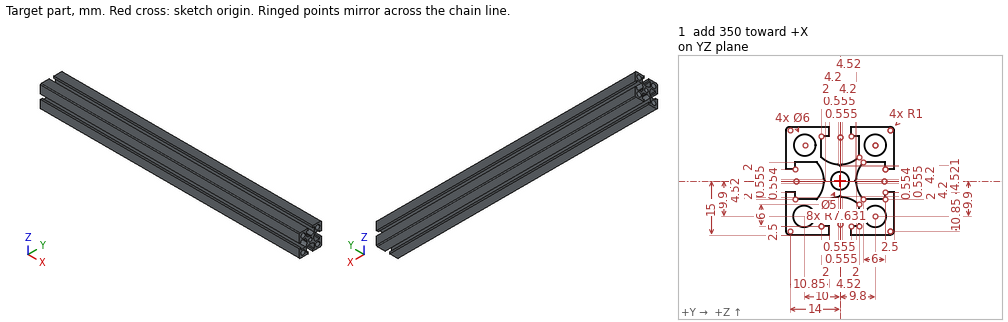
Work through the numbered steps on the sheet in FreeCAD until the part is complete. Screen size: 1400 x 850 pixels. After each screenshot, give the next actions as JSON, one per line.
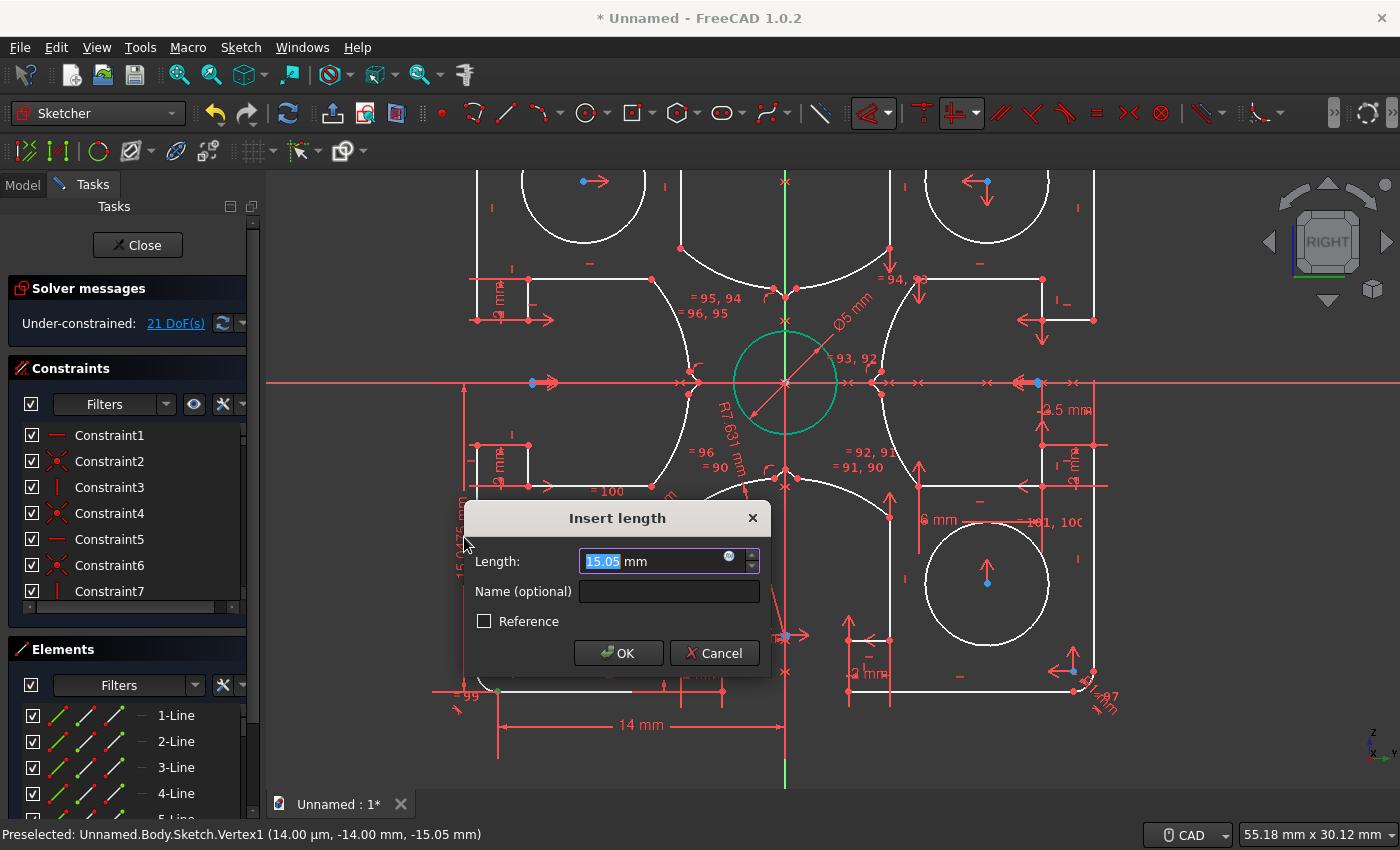
{"action": "type", "text": "15"}
{"action": "key", "text": "Return"}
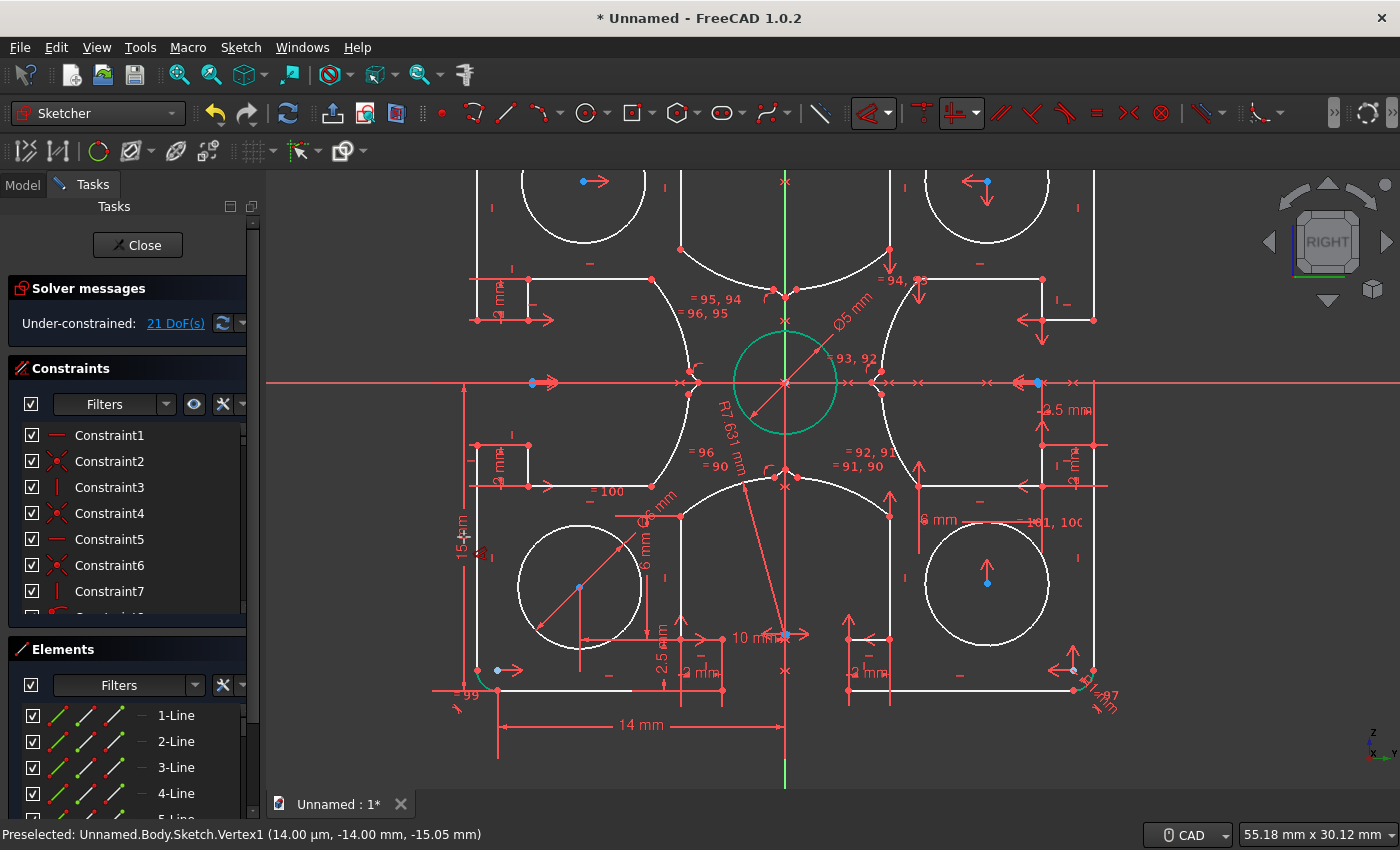
{"action": "left_click", "coordinate": [580, 587]}
{"action": "left_click", "coordinate": [546, 438]}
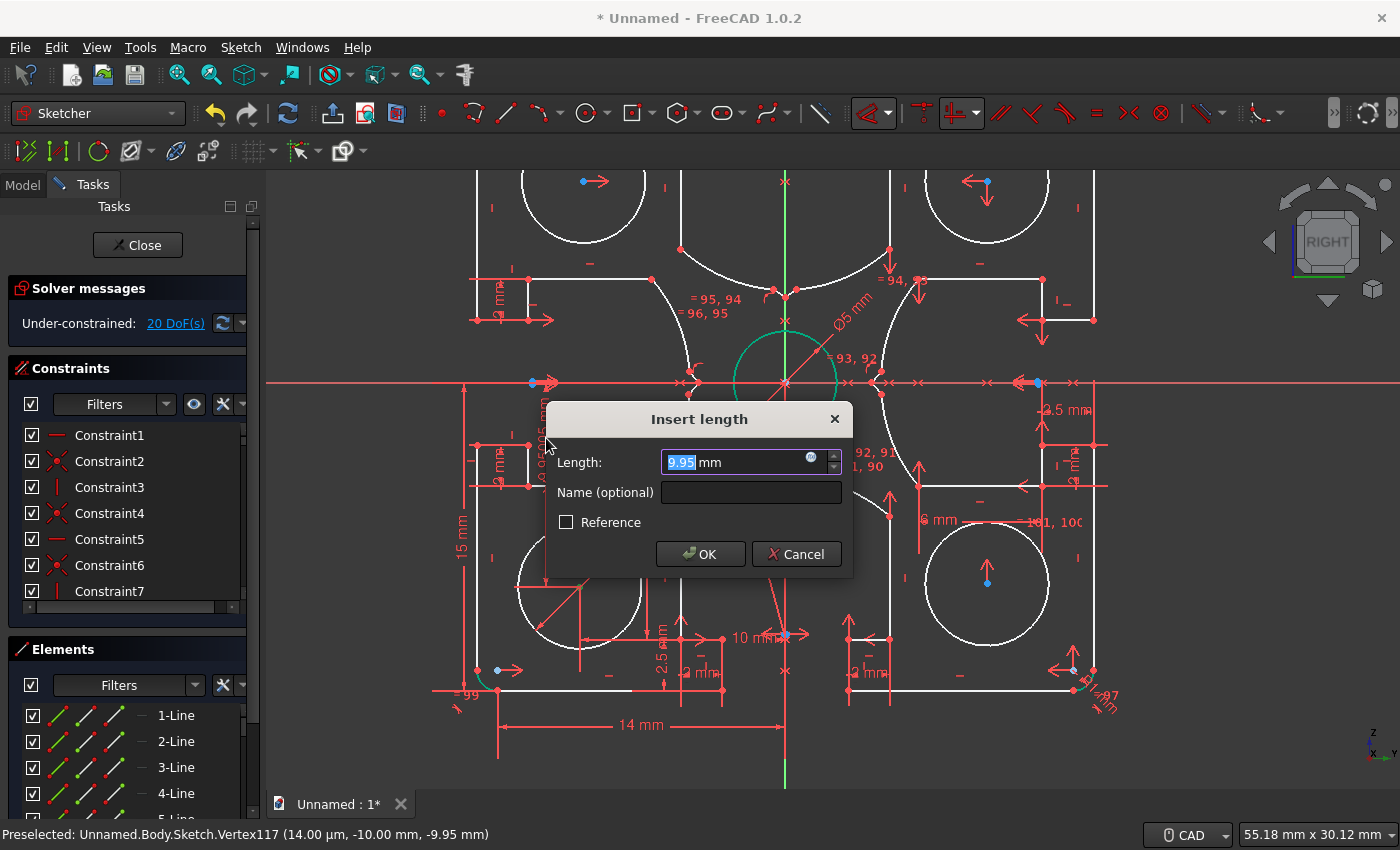
{"action": "type", "text": "9.9"}
{"action": "key", "text": "Return"}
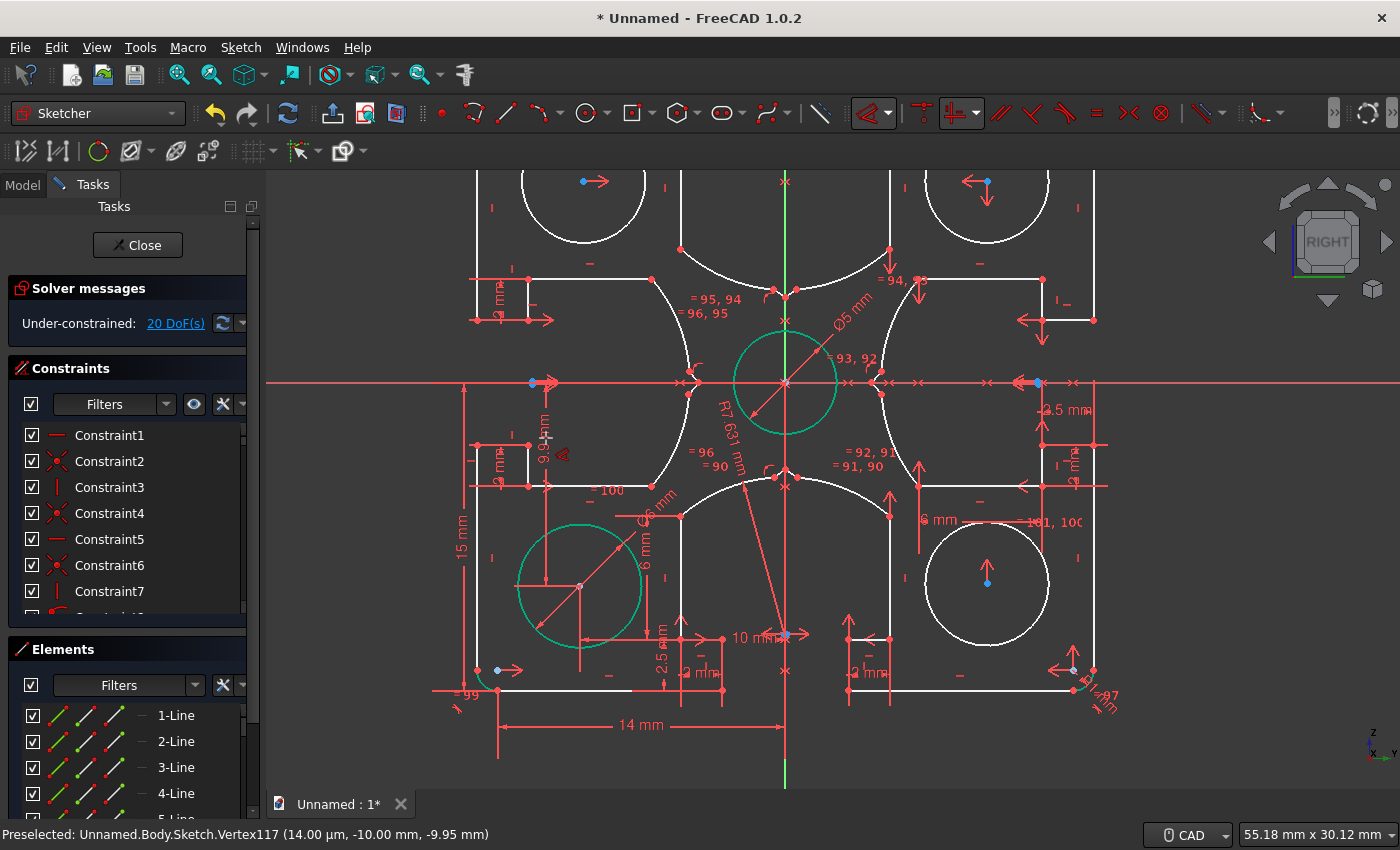
{"action": "left_click", "coordinate": [987, 584]}
{"action": "left_click", "coordinate": [840, 618]}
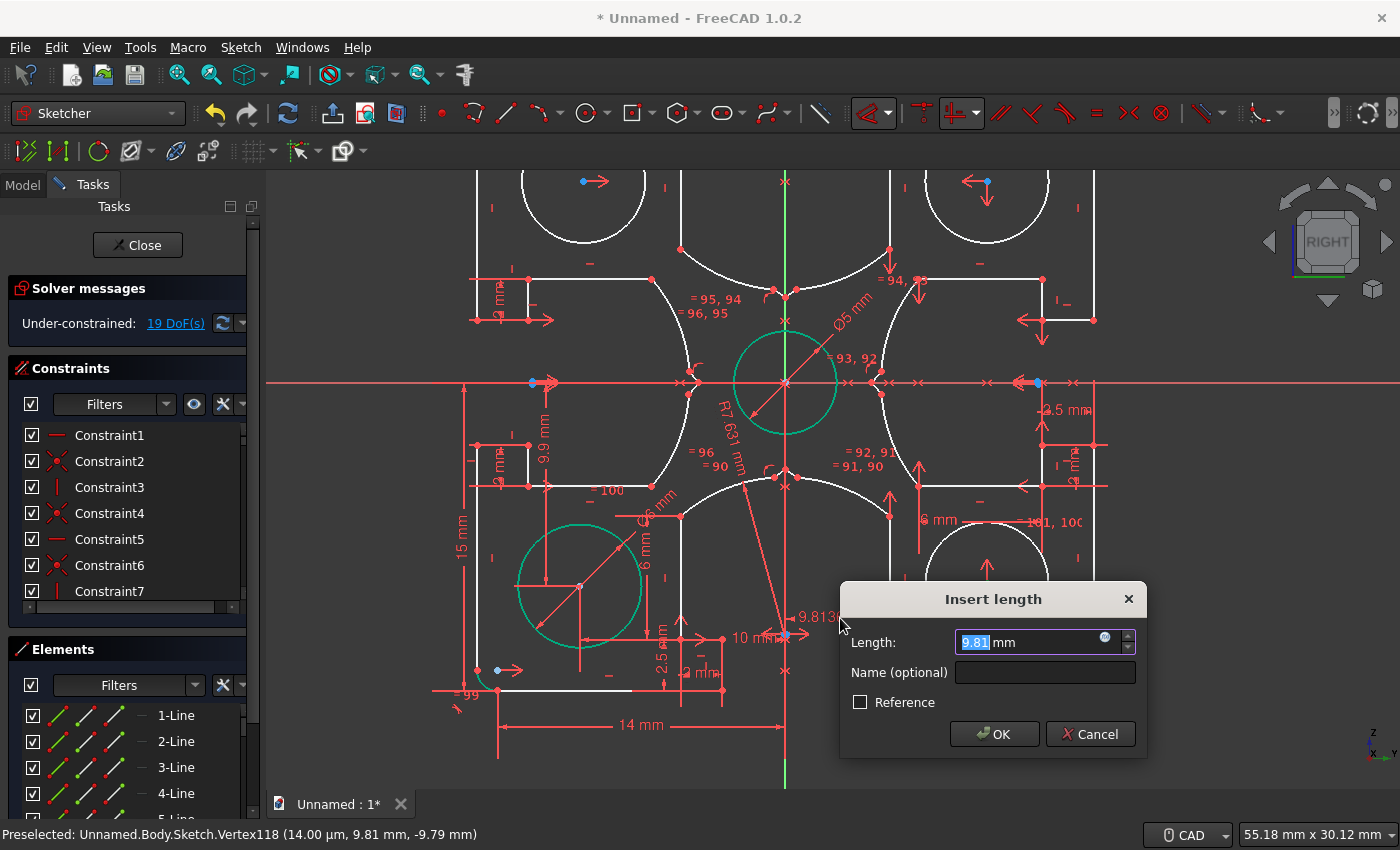
{"action": "type", "text": "9.8"}
{"action": "key", "text": "Return"}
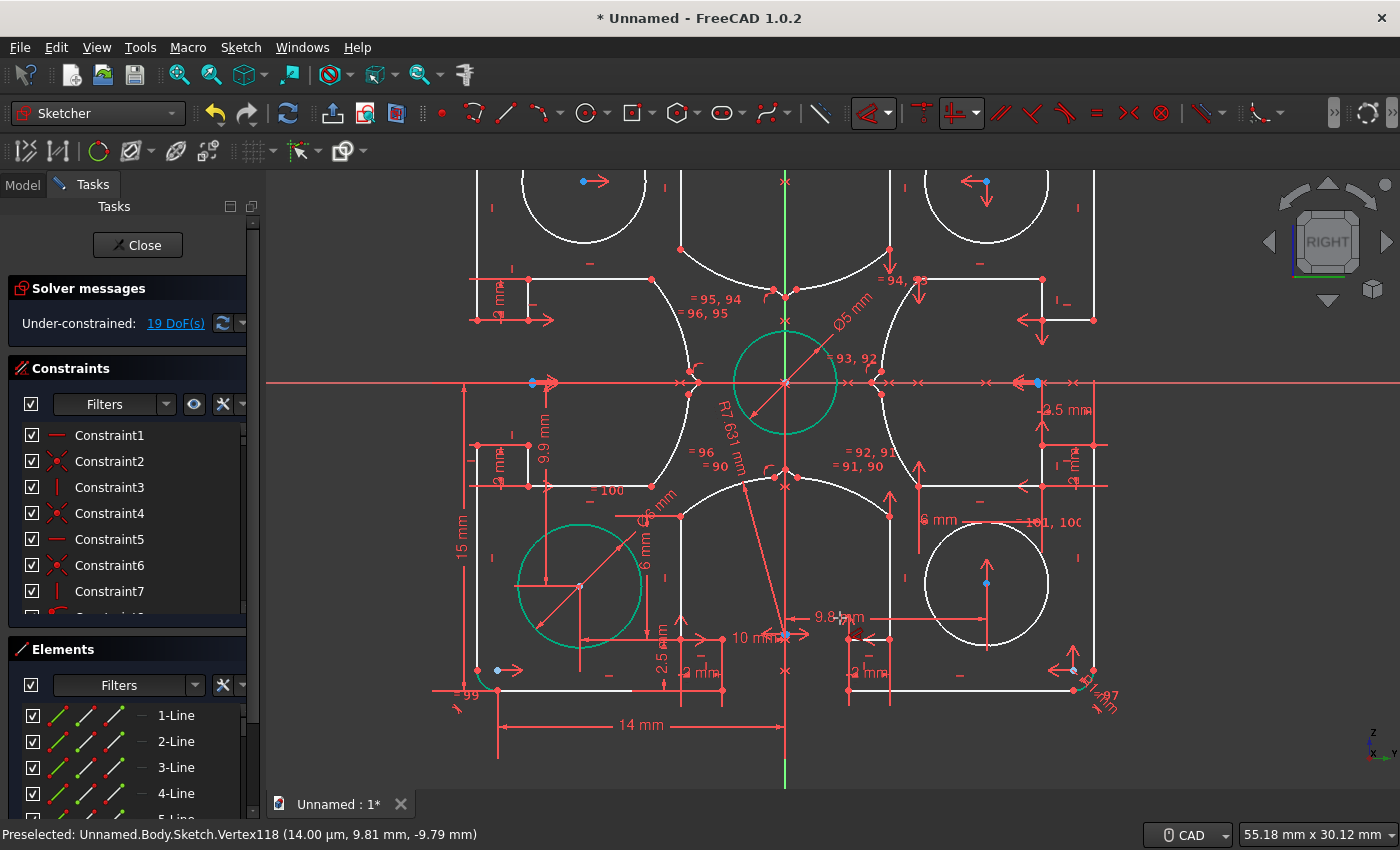
{"action": "left_click", "coordinate": [987, 584]}
{"action": "left_click", "coordinate": [1021, 437]}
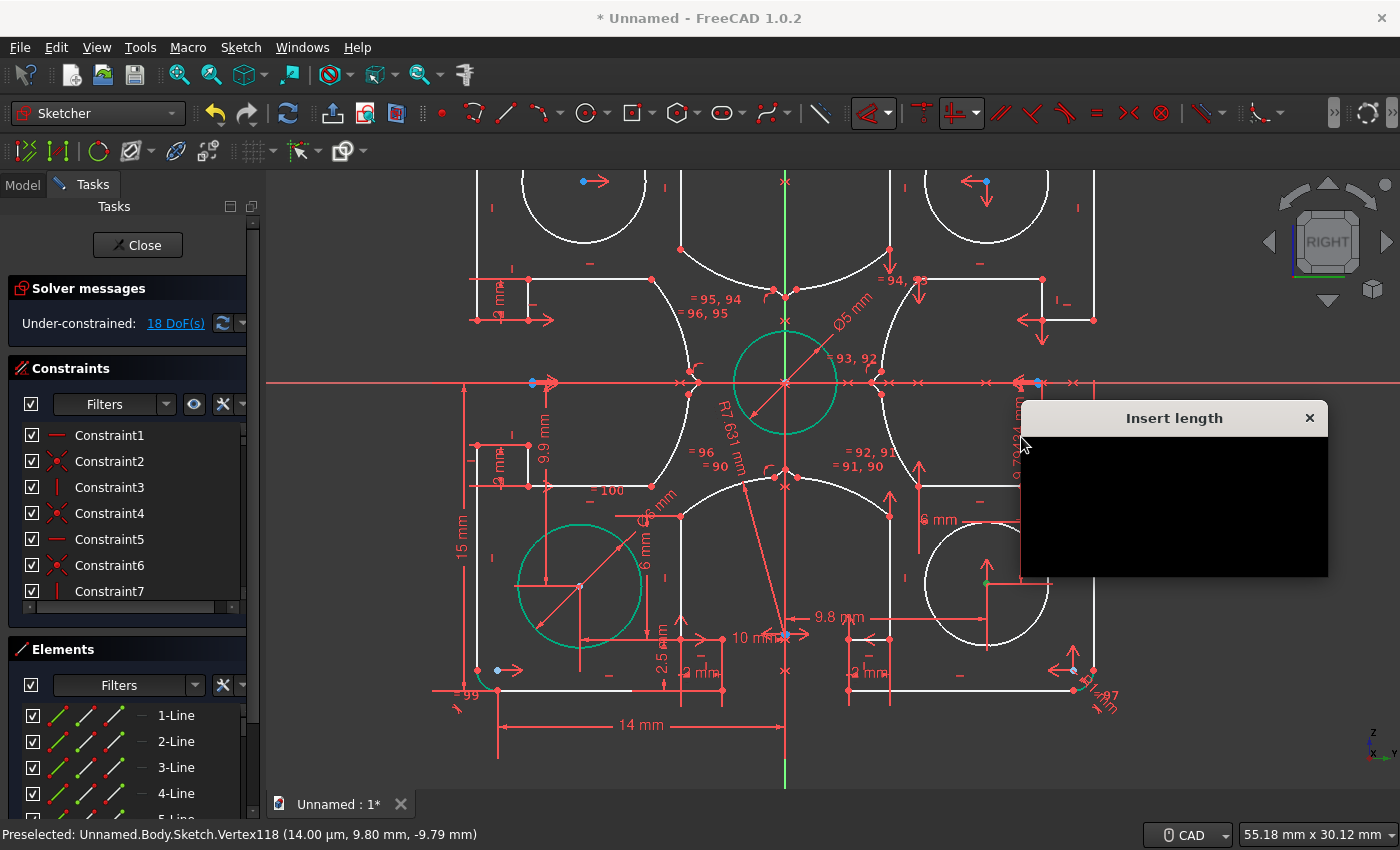
{"action": "type", "text": "9.9"}
{"action": "key", "text": "Return"}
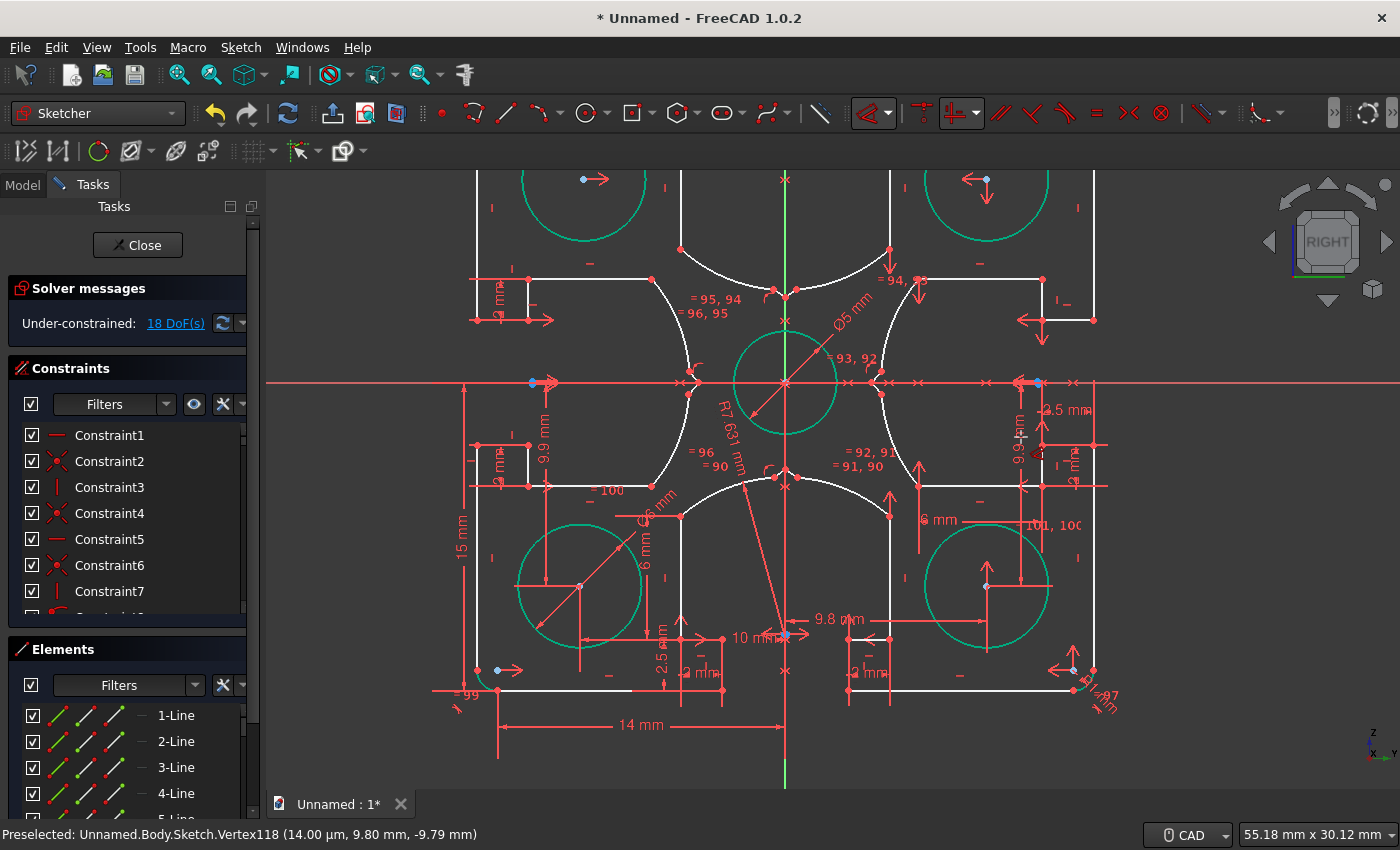
{"action": "left_click", "coordinate": [785, 469]}
{"action": "left_click", "coordinate": [819, 446]}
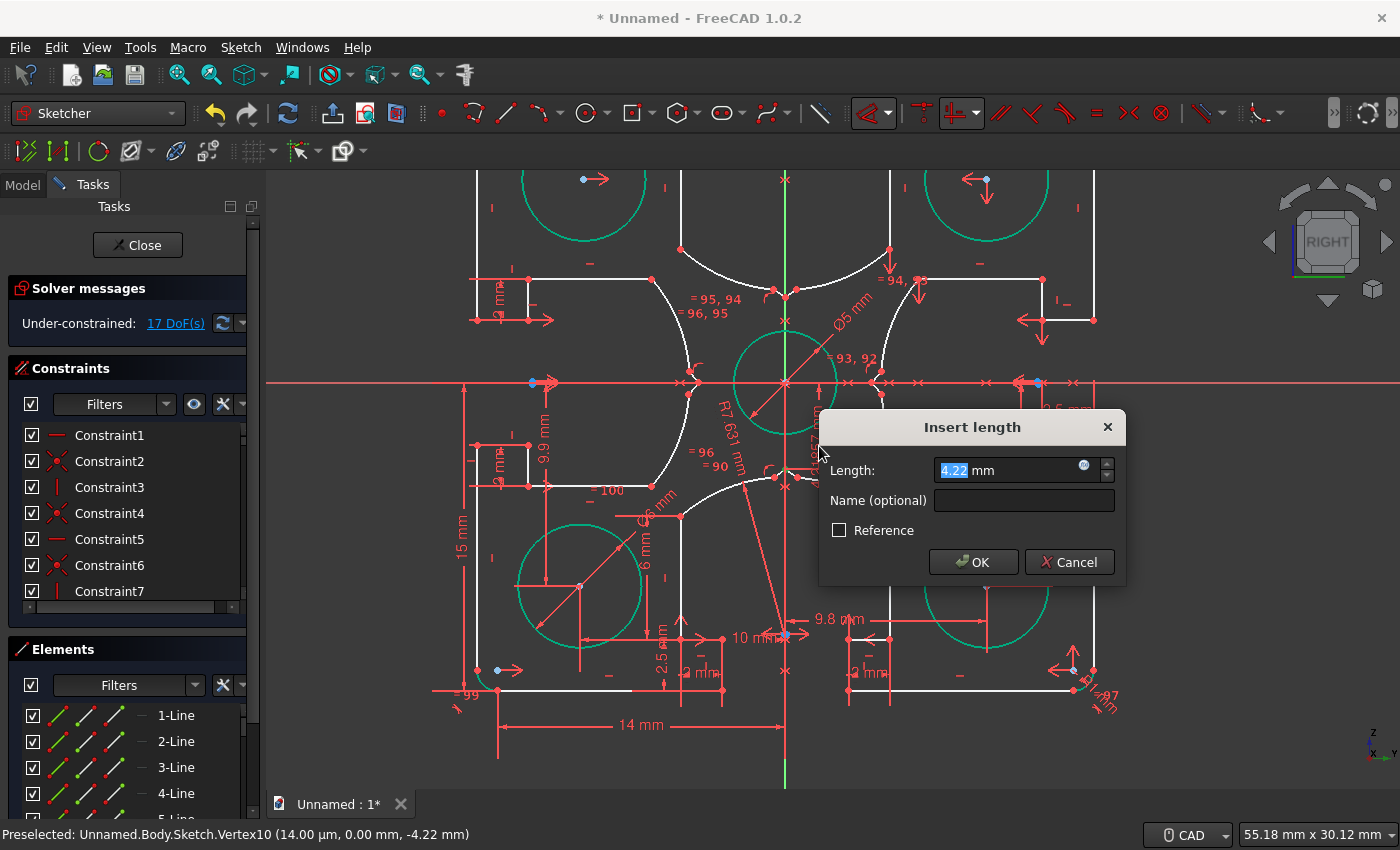
{"action": "type", "text": "4.2"}
{"action": "key", "text": "Return"}